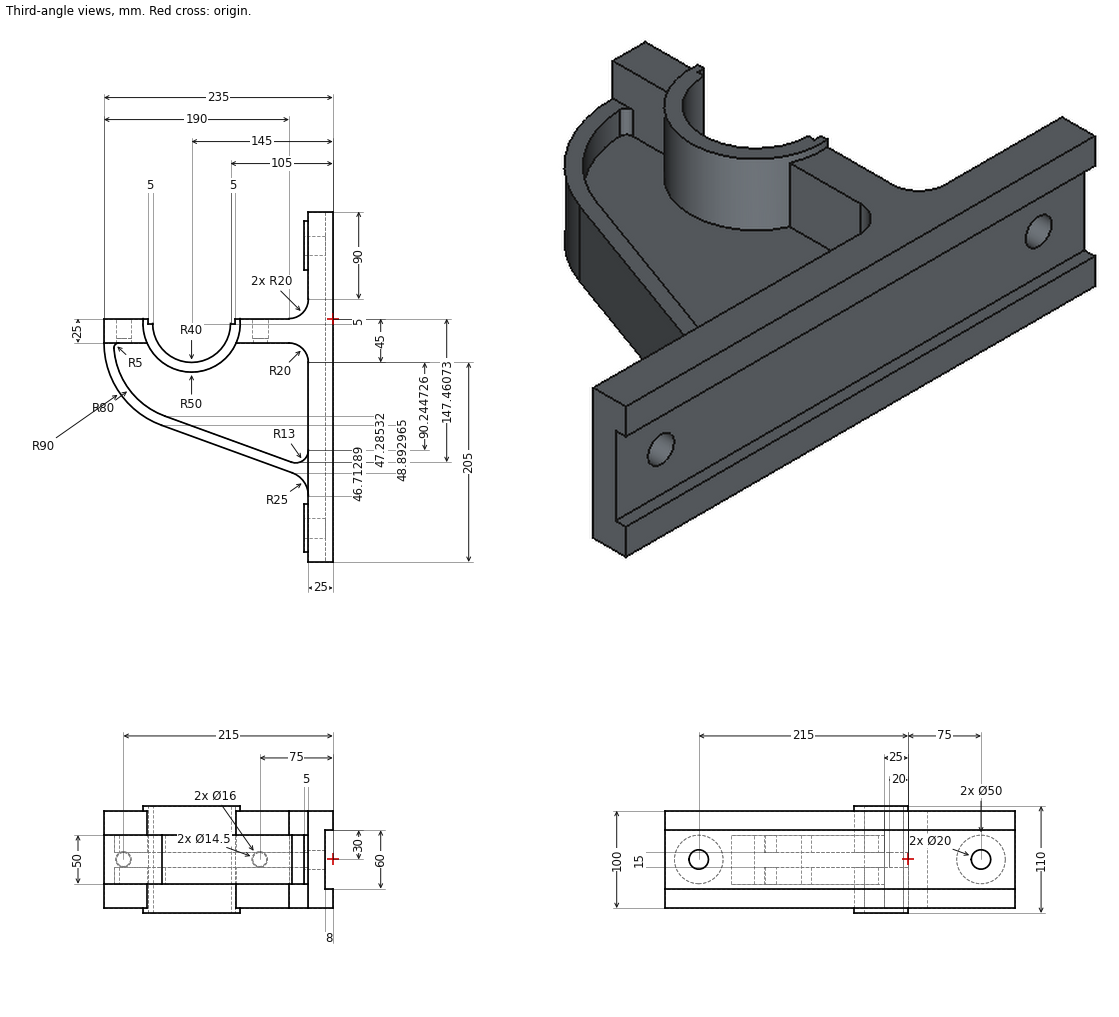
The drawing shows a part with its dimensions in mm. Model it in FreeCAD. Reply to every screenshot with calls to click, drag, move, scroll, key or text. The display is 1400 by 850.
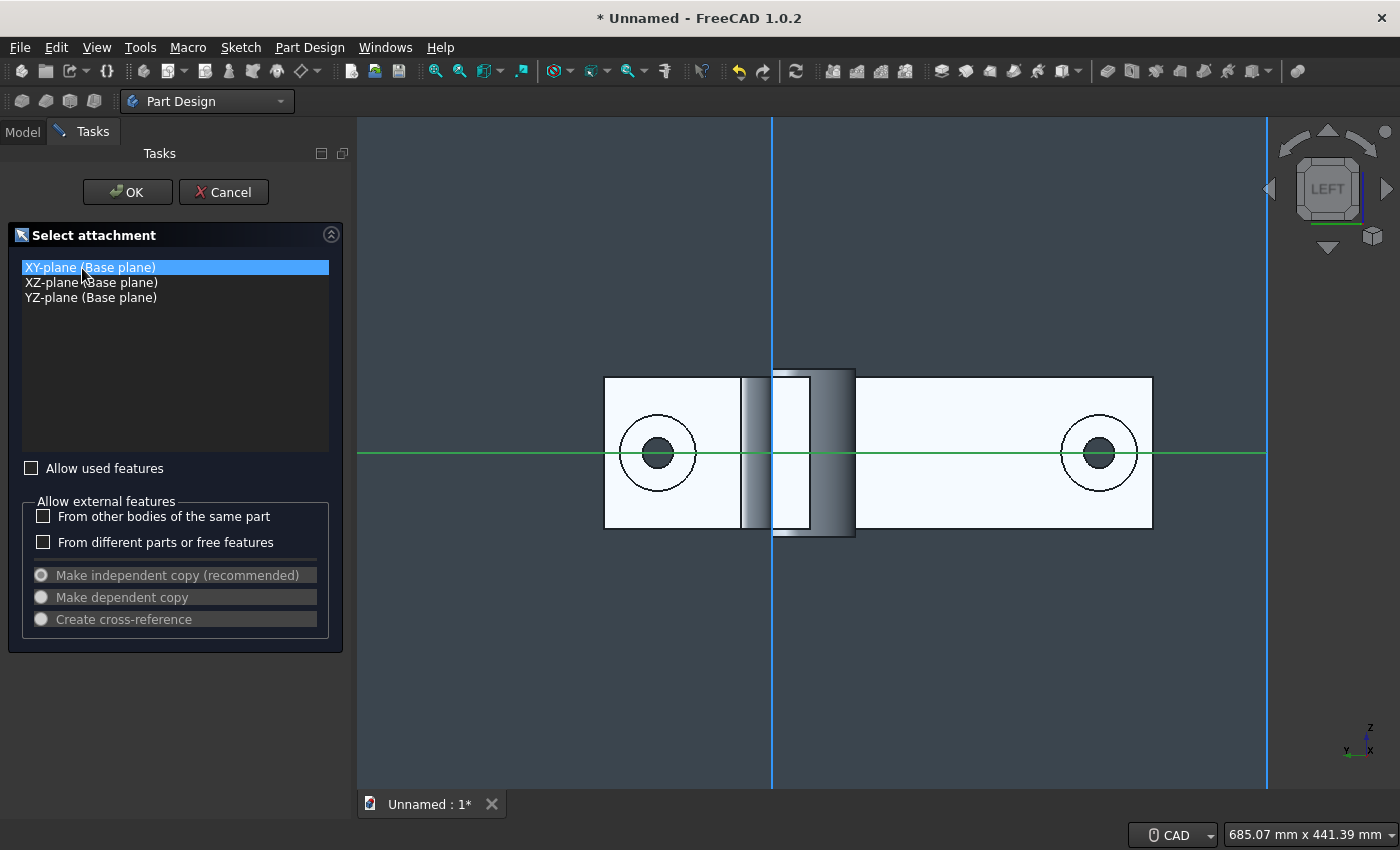
click(128, 192)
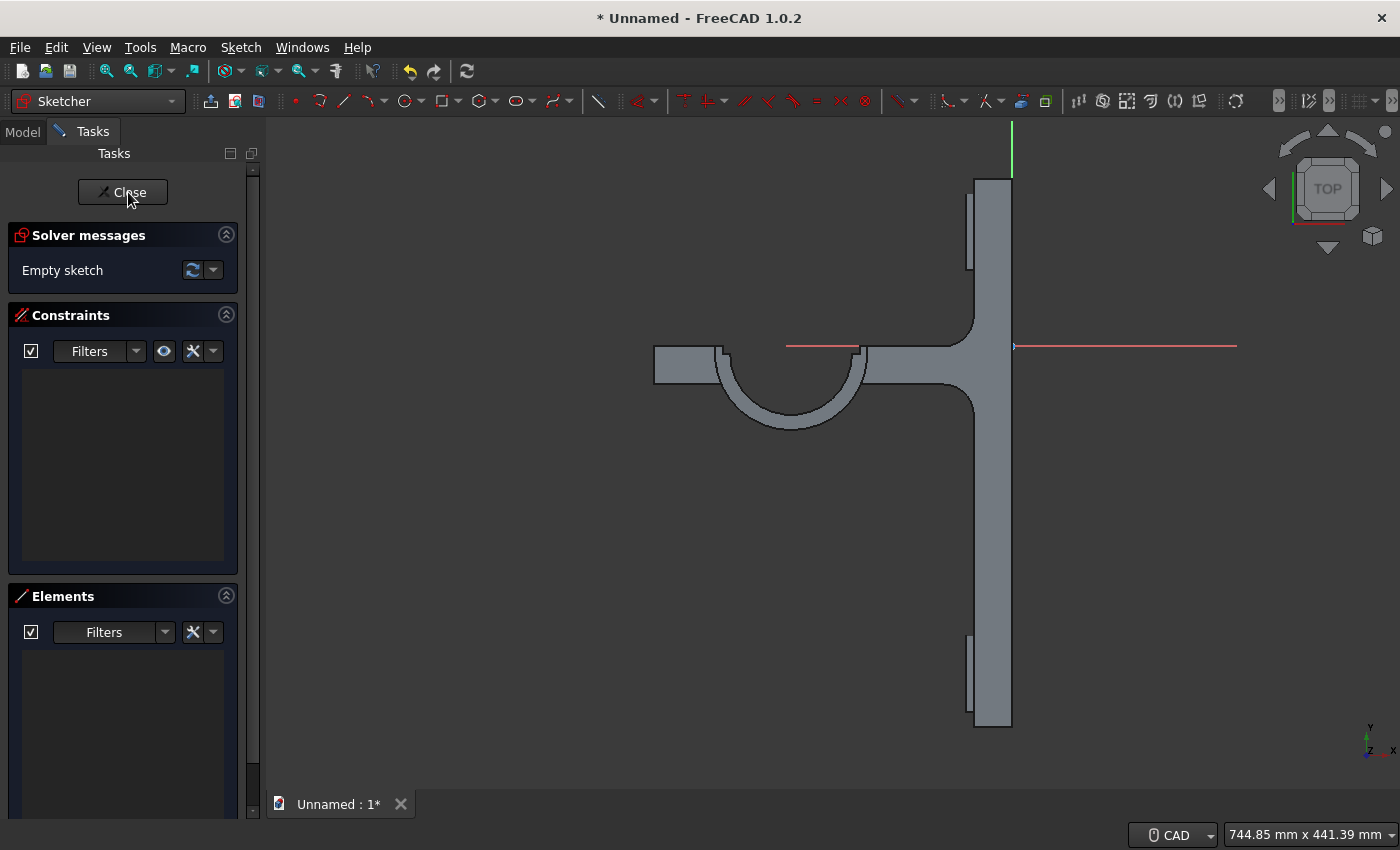
click(260, 102)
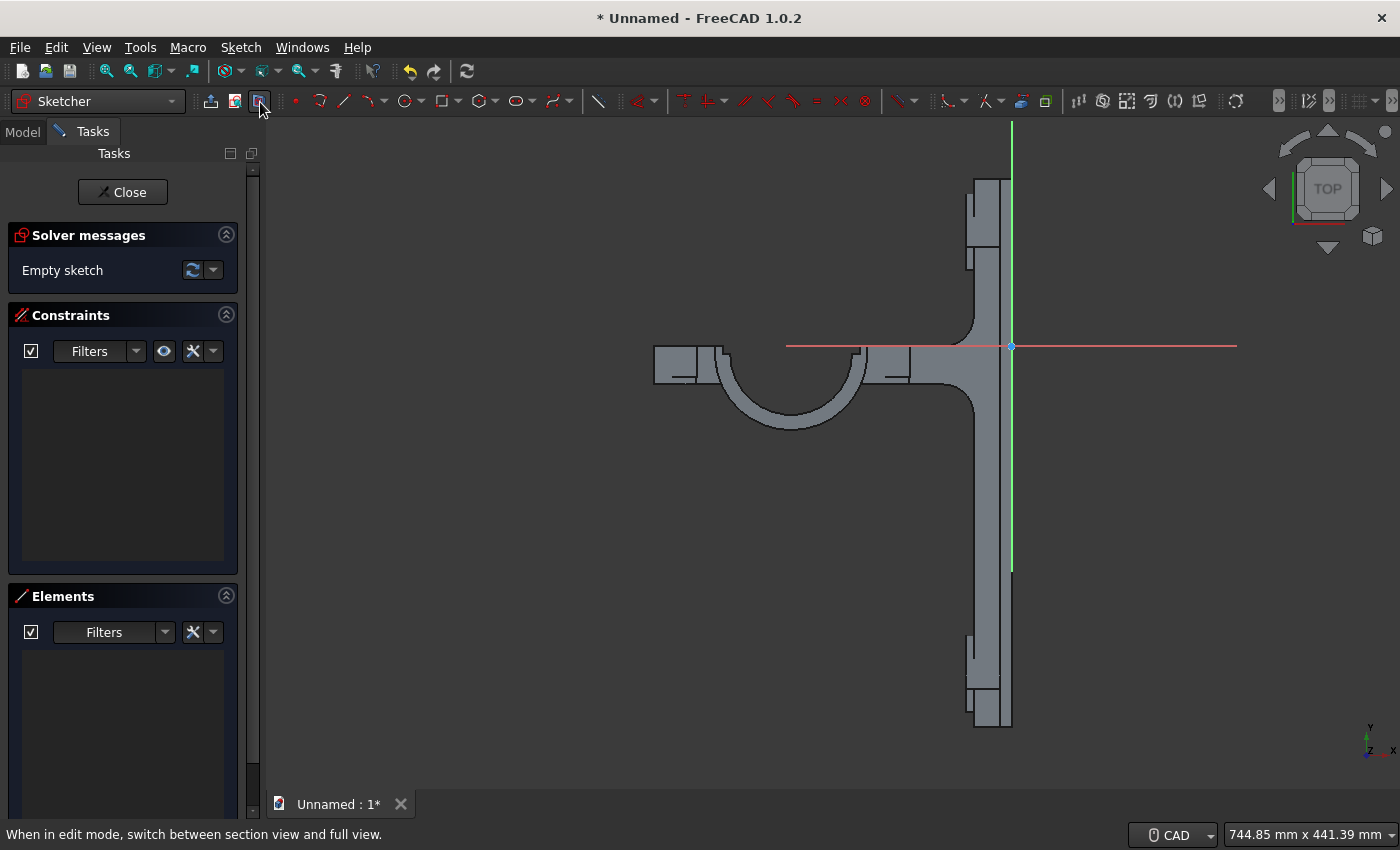
scroll(972, 550, up, 2)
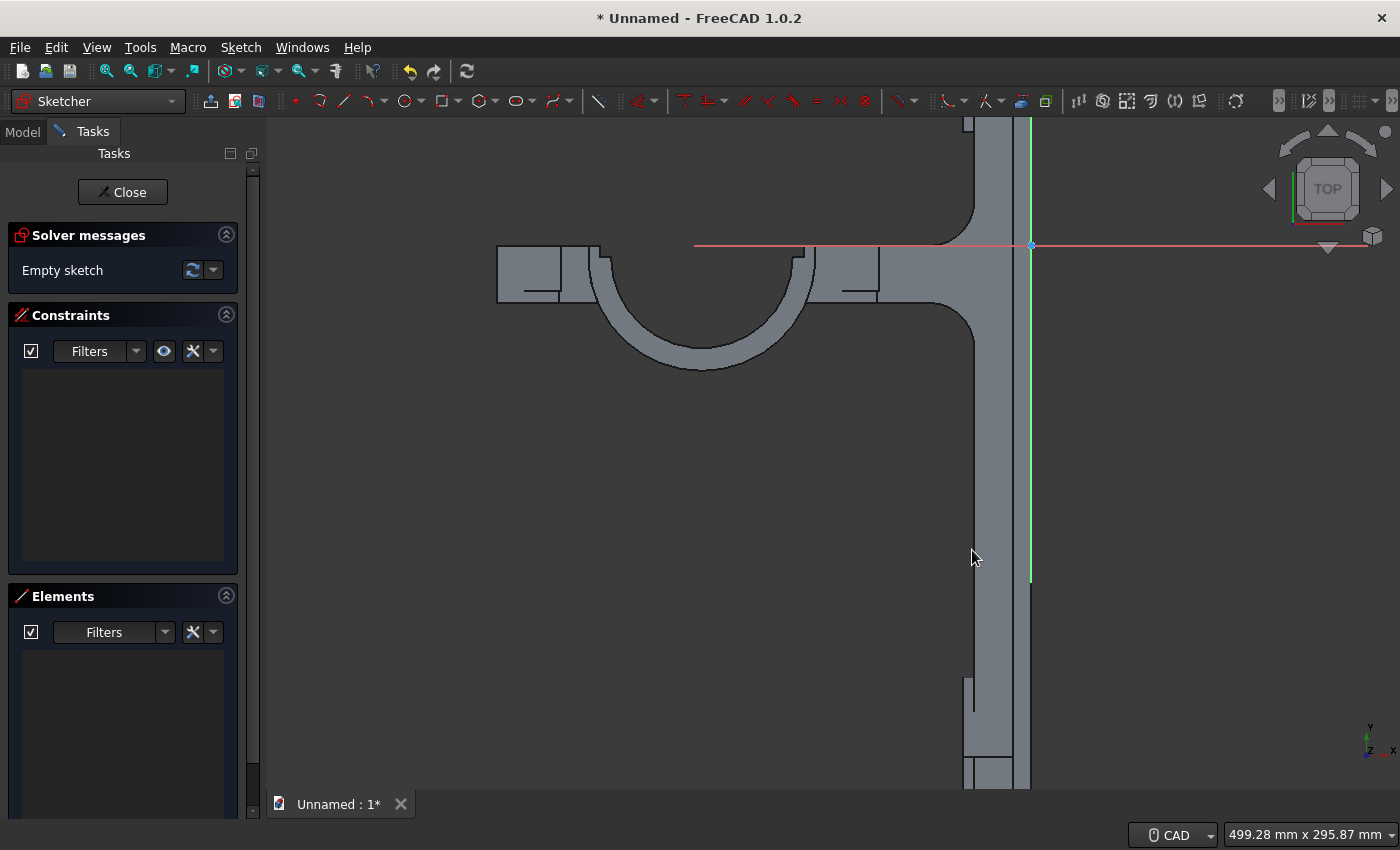
click(344, 102)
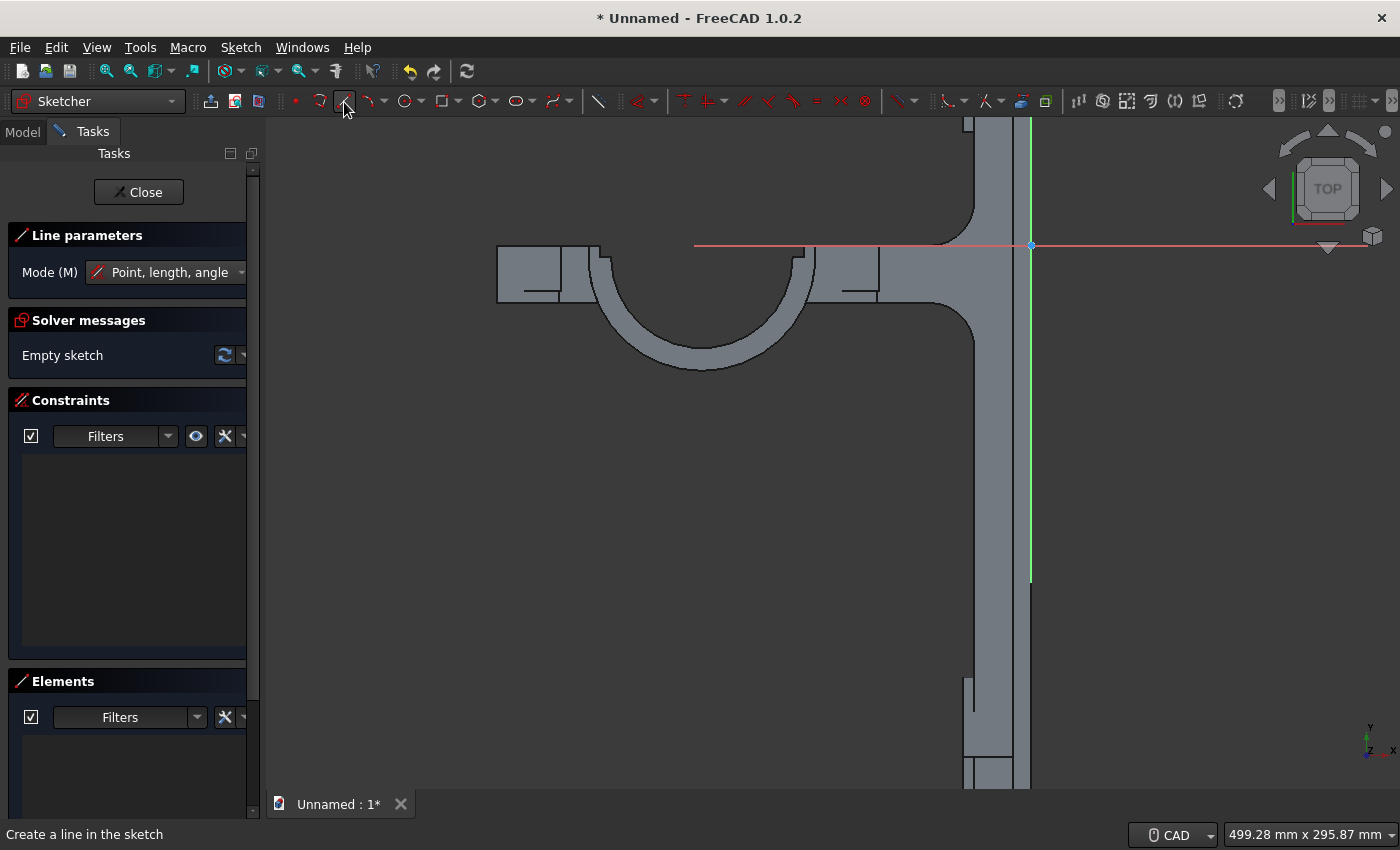
click(632, 495)
click(937, 606)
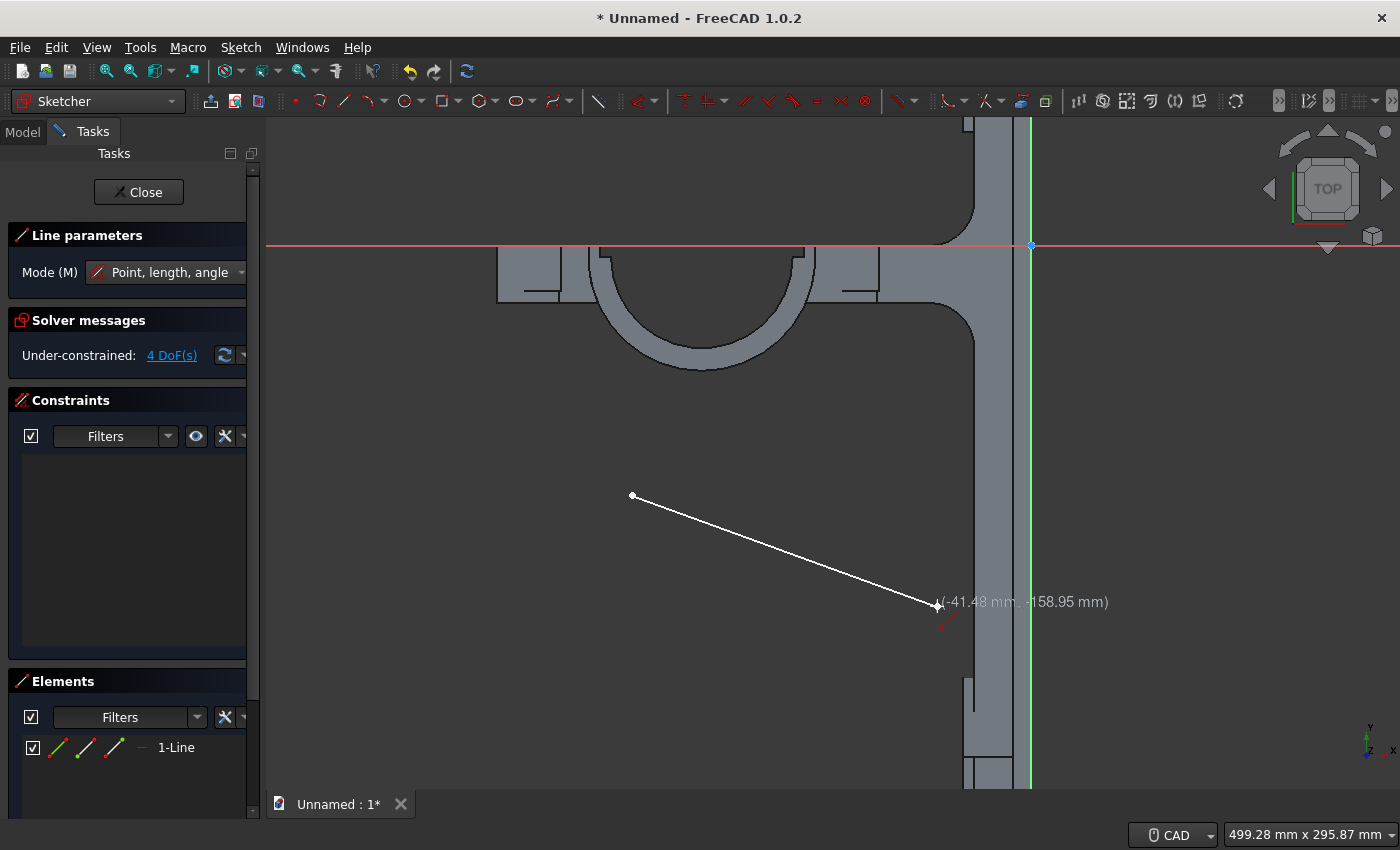
click(974, 659)
click(974, 553)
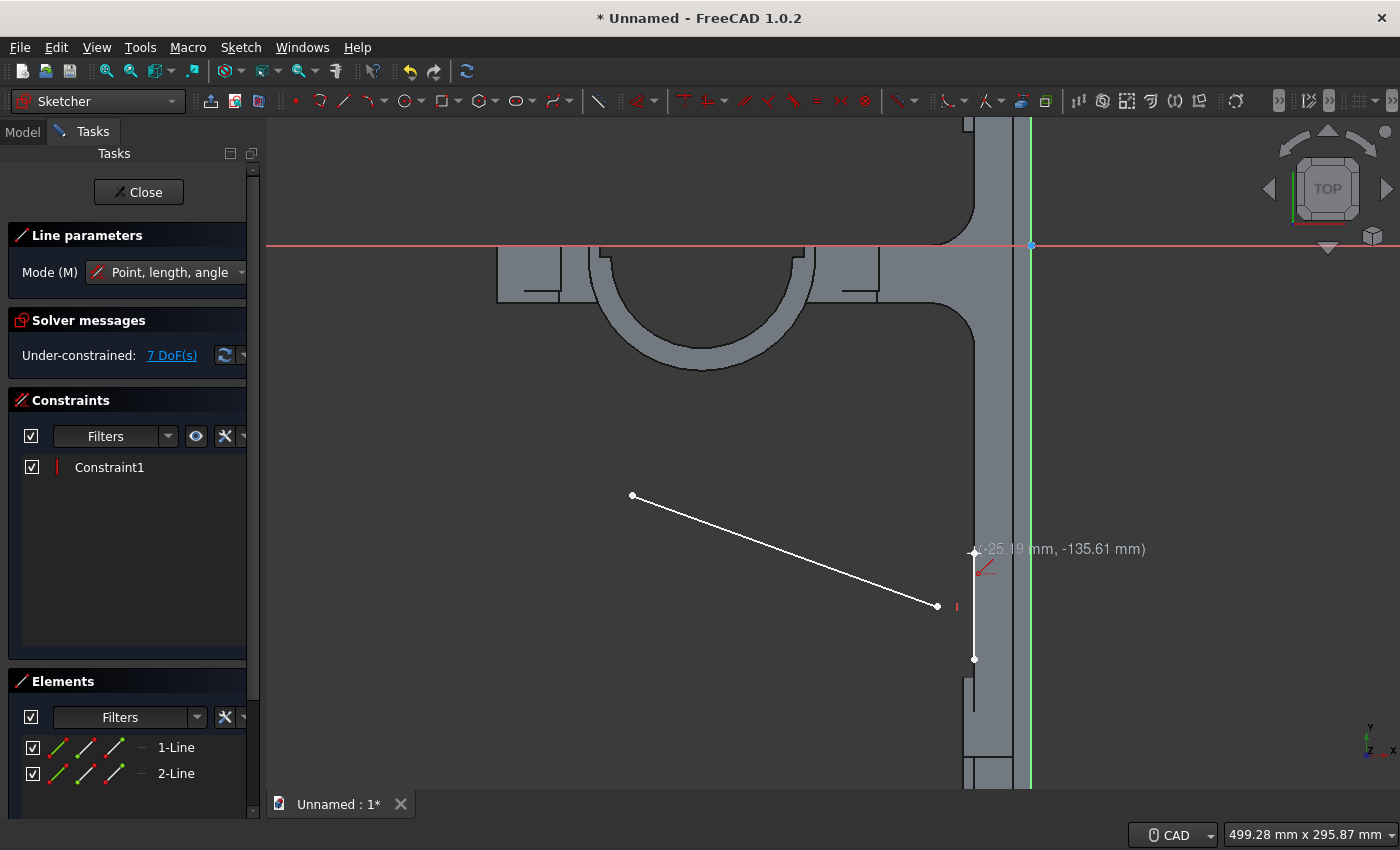
click(935, 581)
click(640, 474)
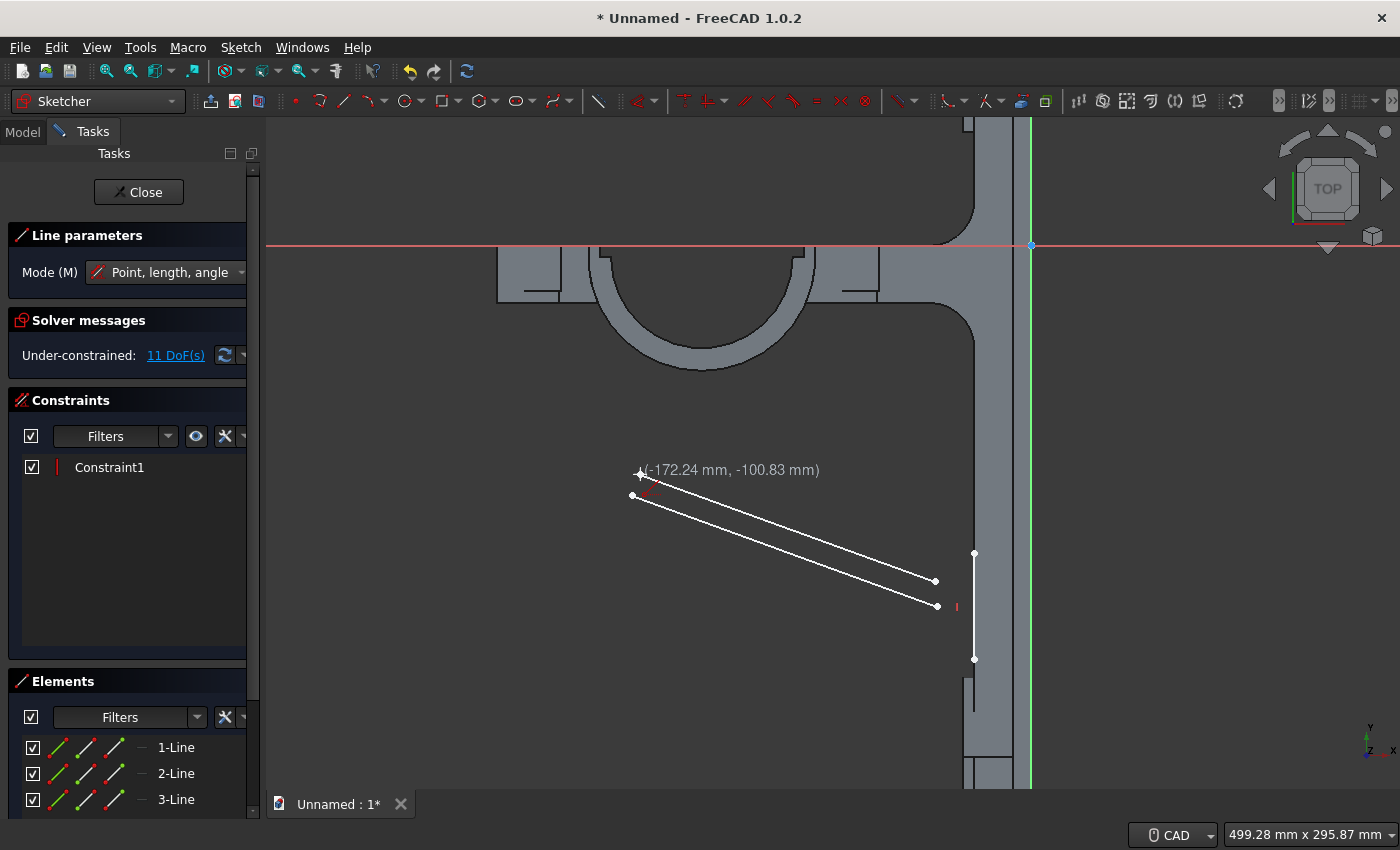
click(532, 303)
click(497, 303)